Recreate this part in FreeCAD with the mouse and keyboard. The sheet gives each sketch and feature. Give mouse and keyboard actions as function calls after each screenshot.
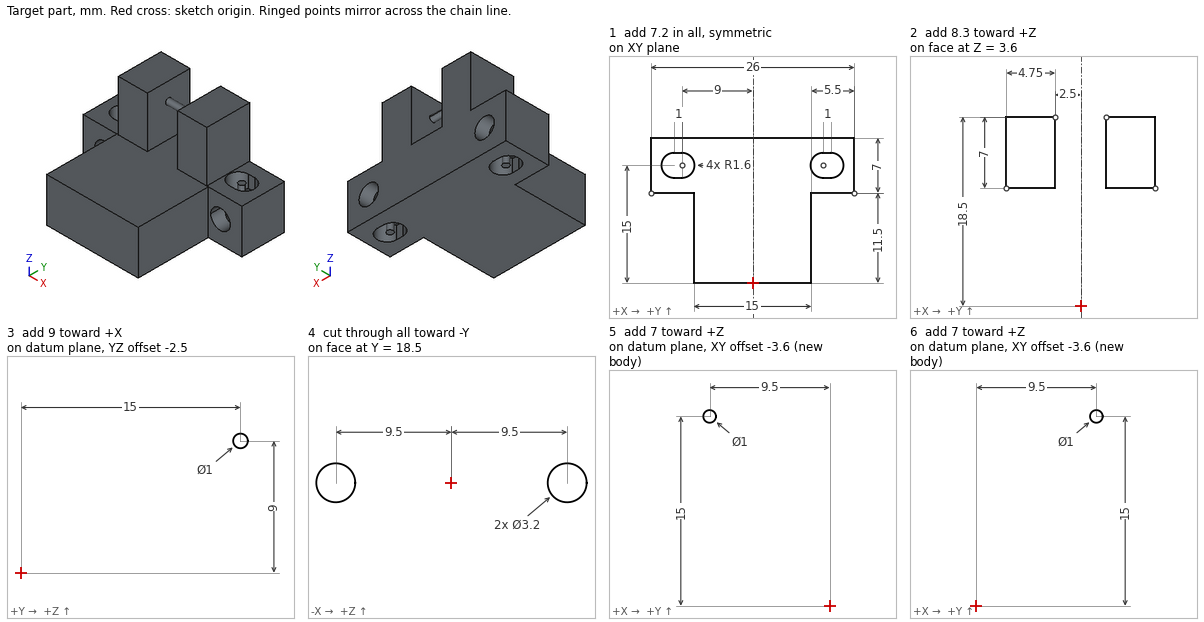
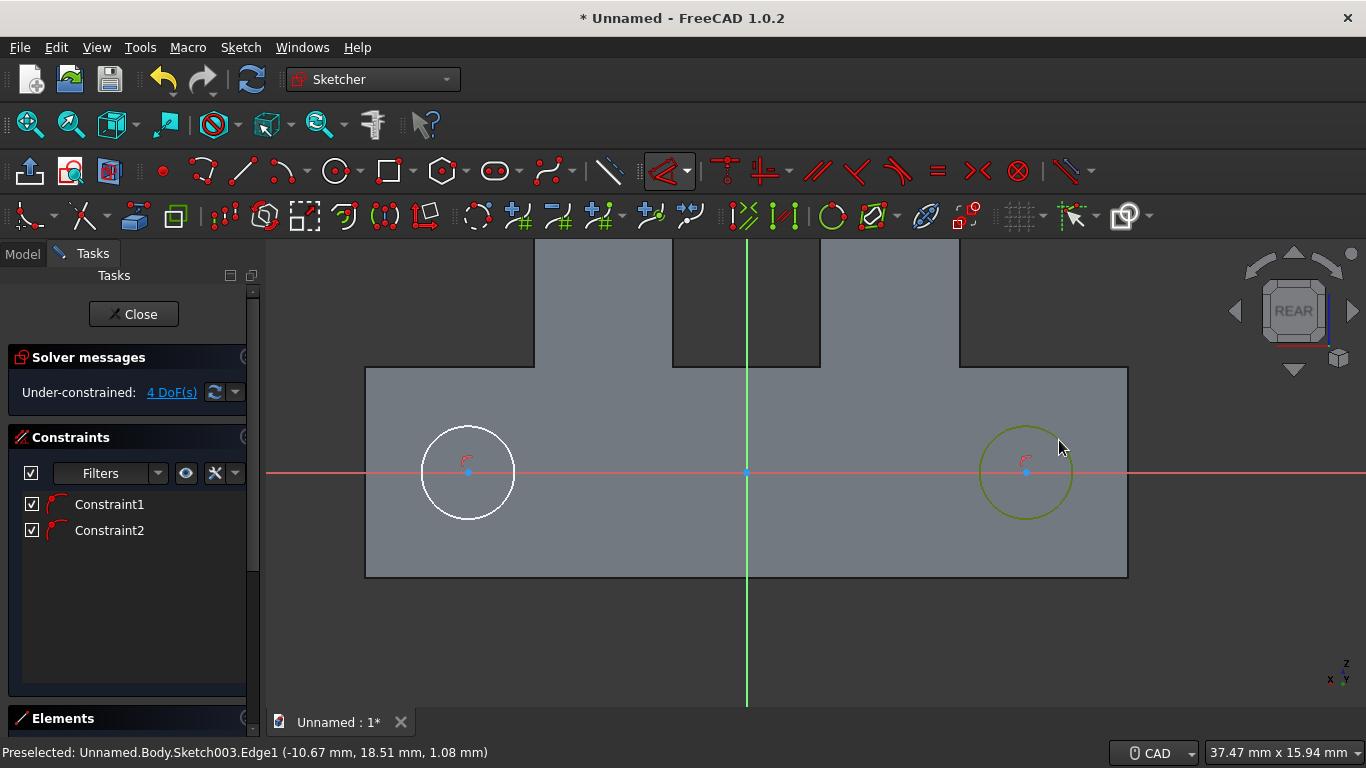
click(501, 440)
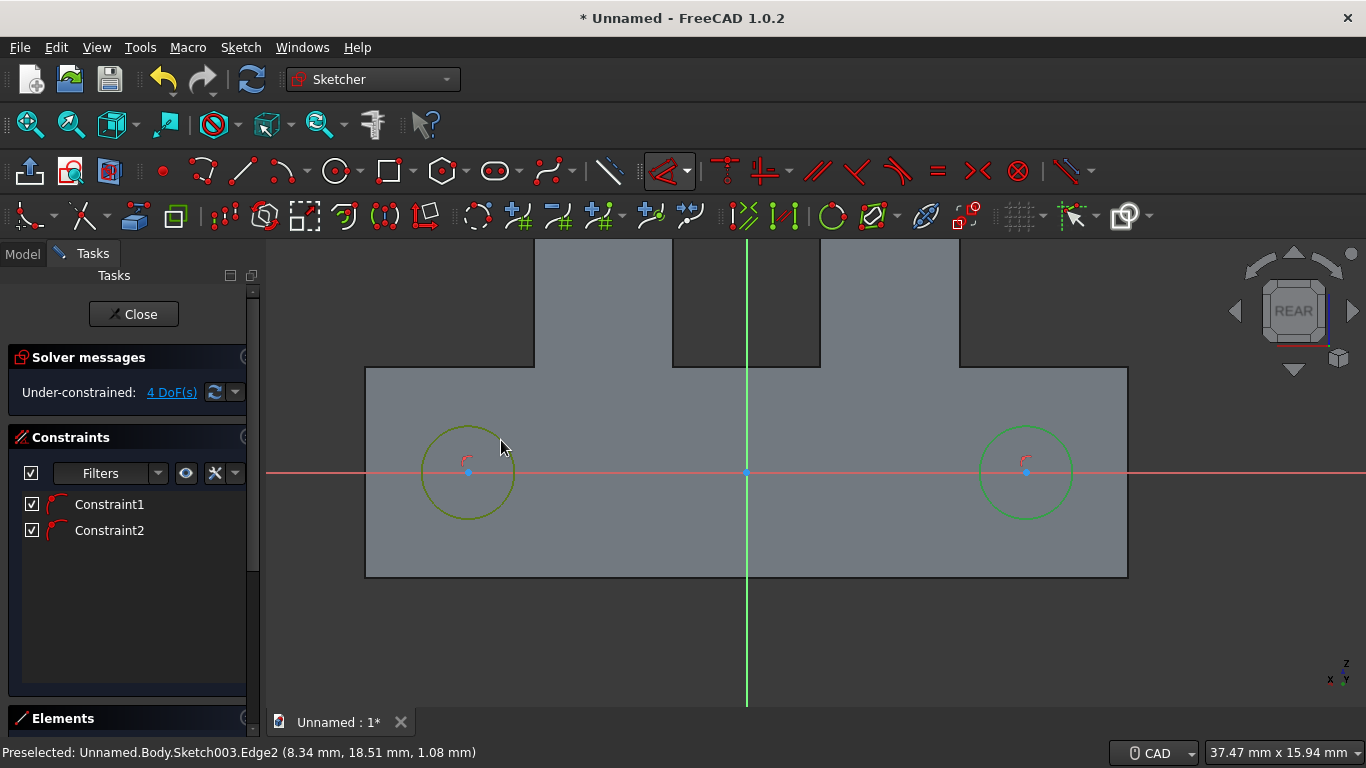
key(e)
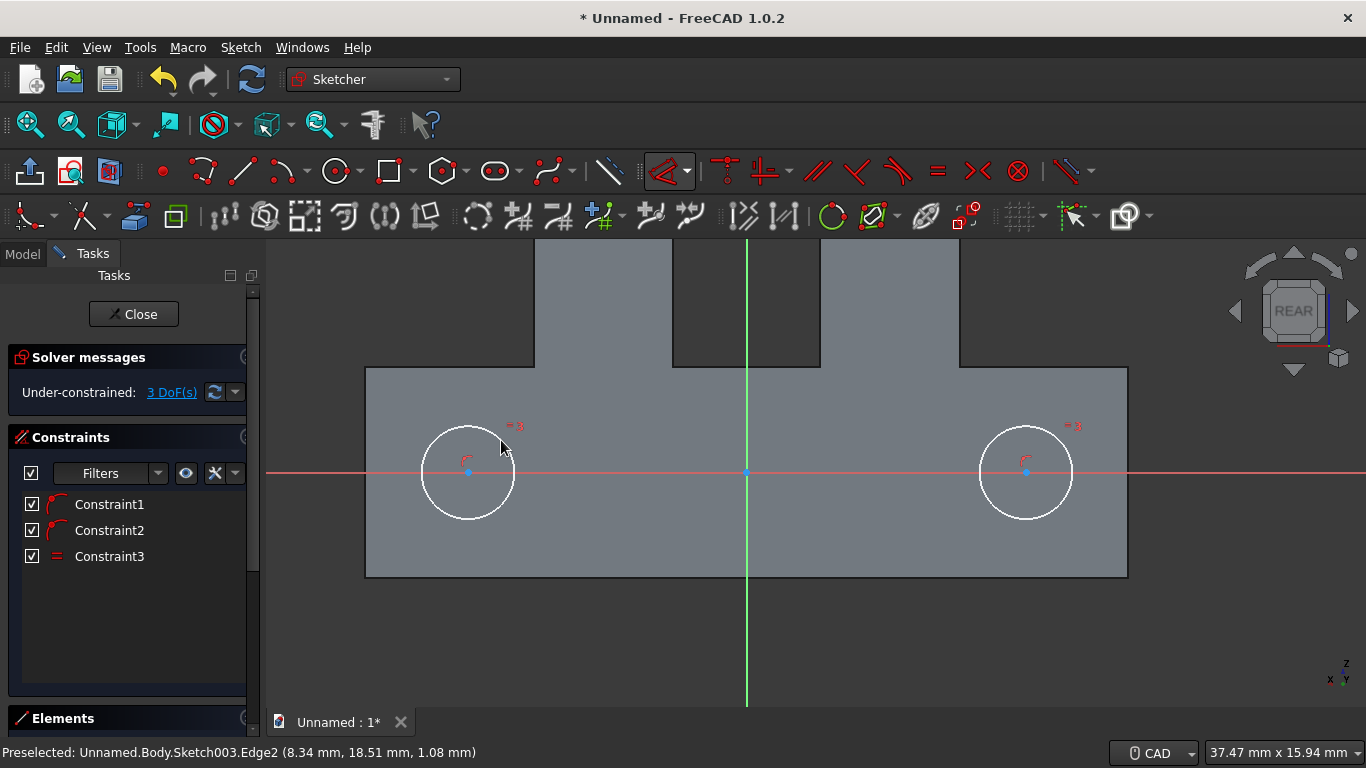
click(1059, 440)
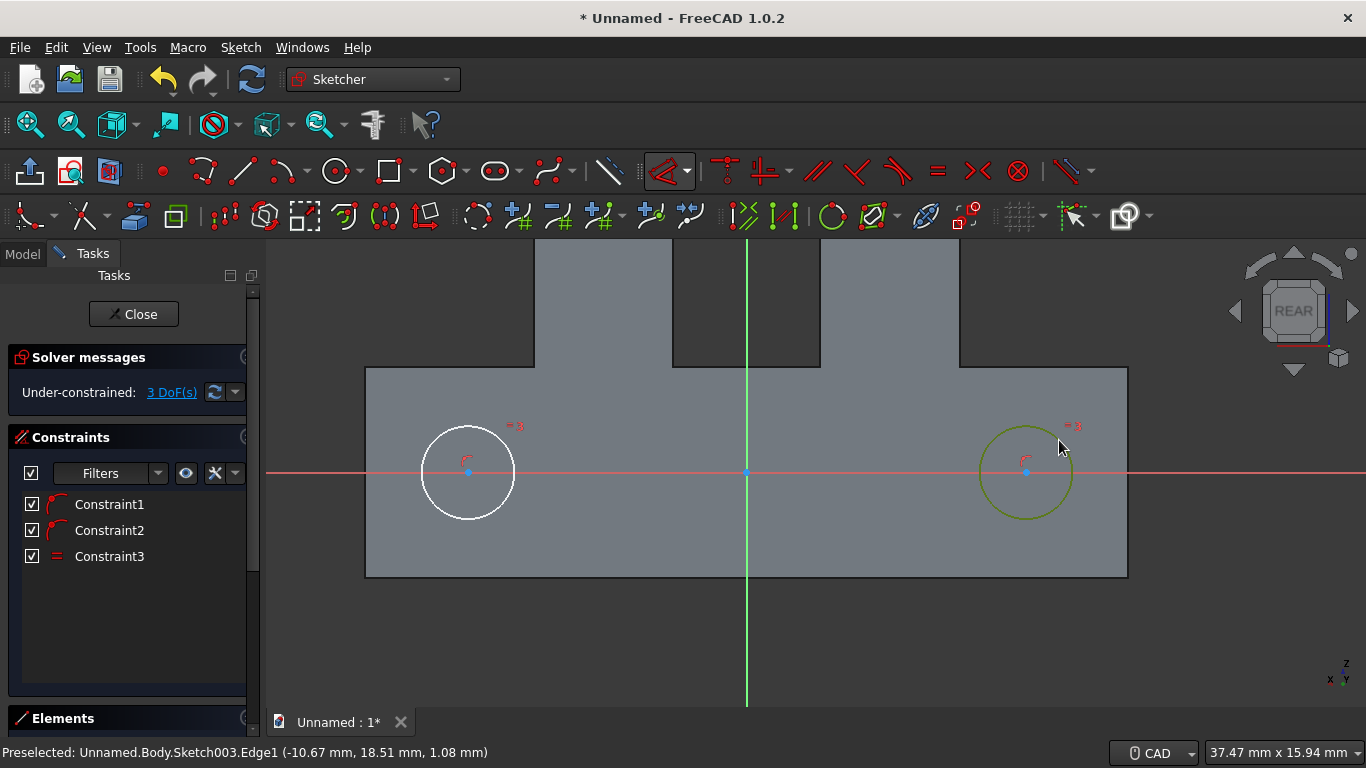
key(k)
key(o)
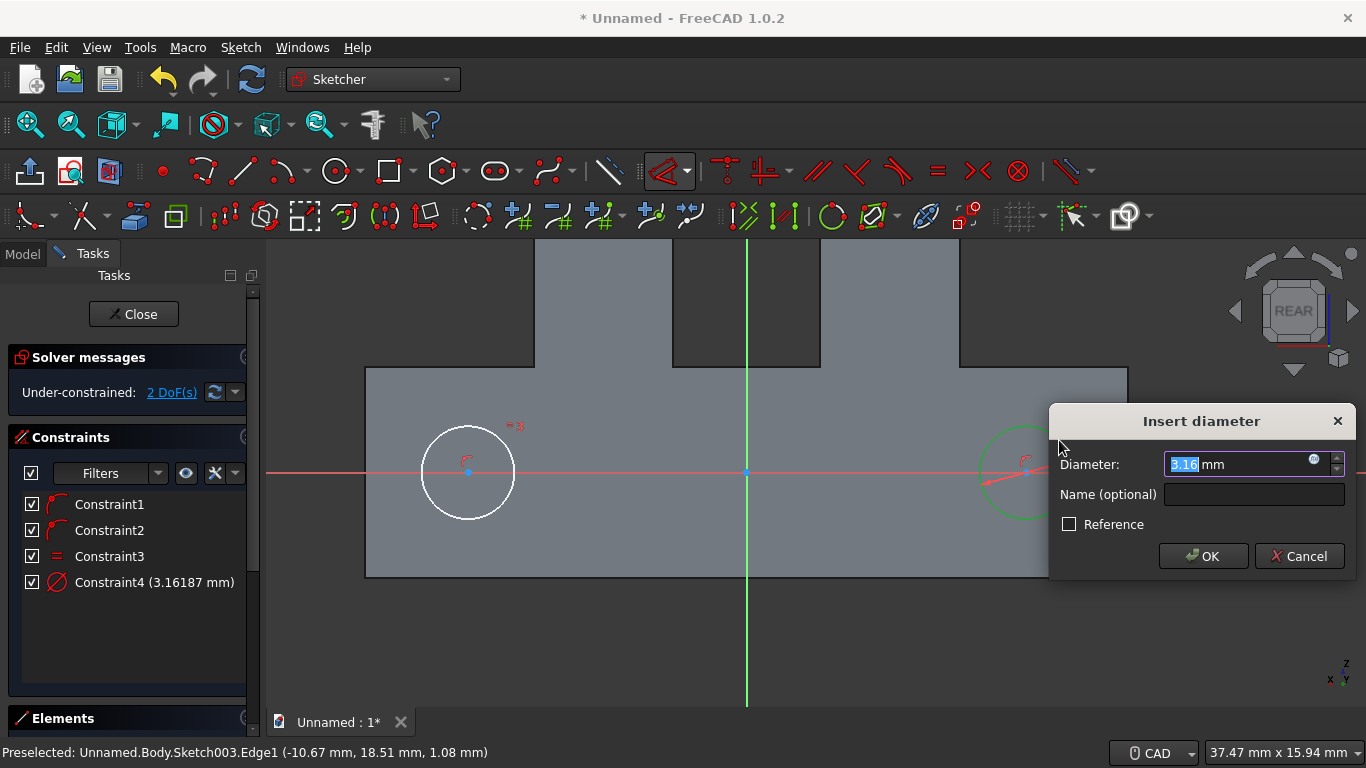
text(3.2)
key(Return)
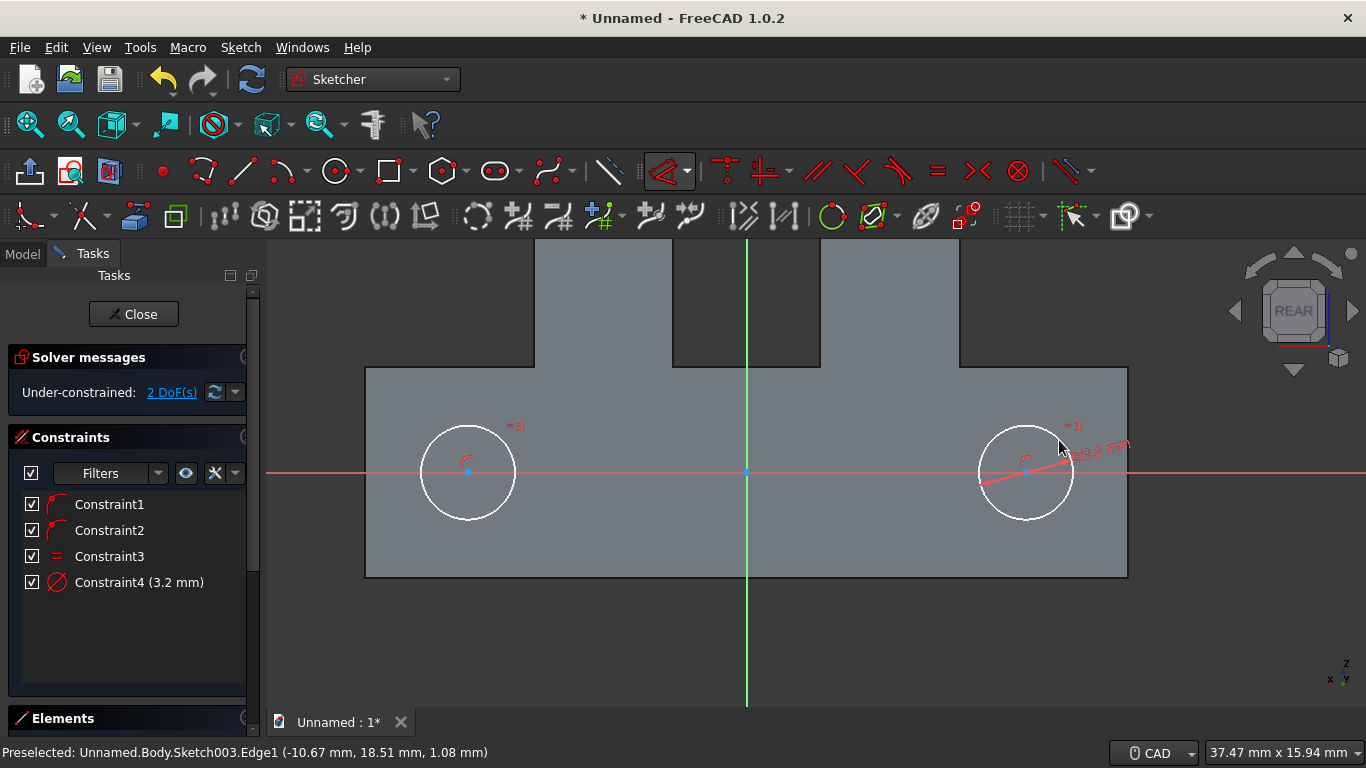
click(1026, 473)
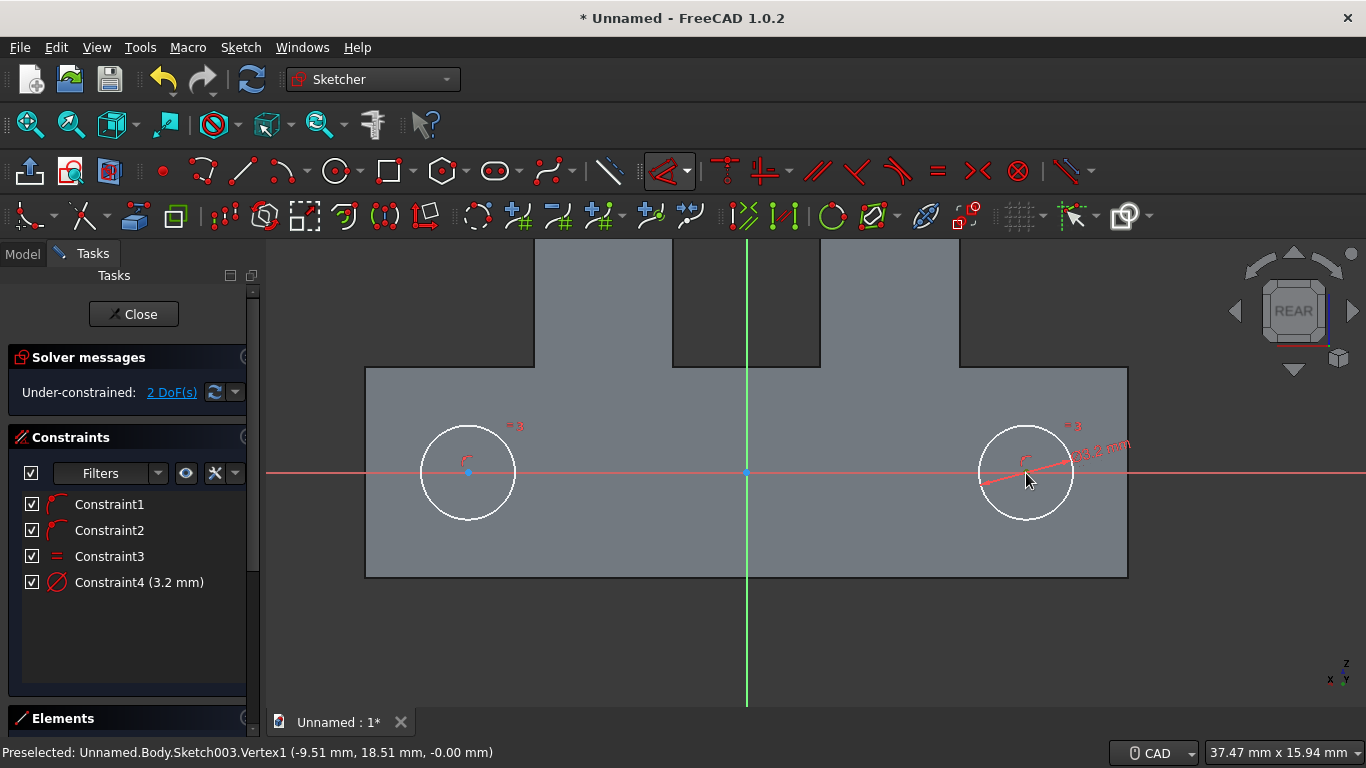
key(l)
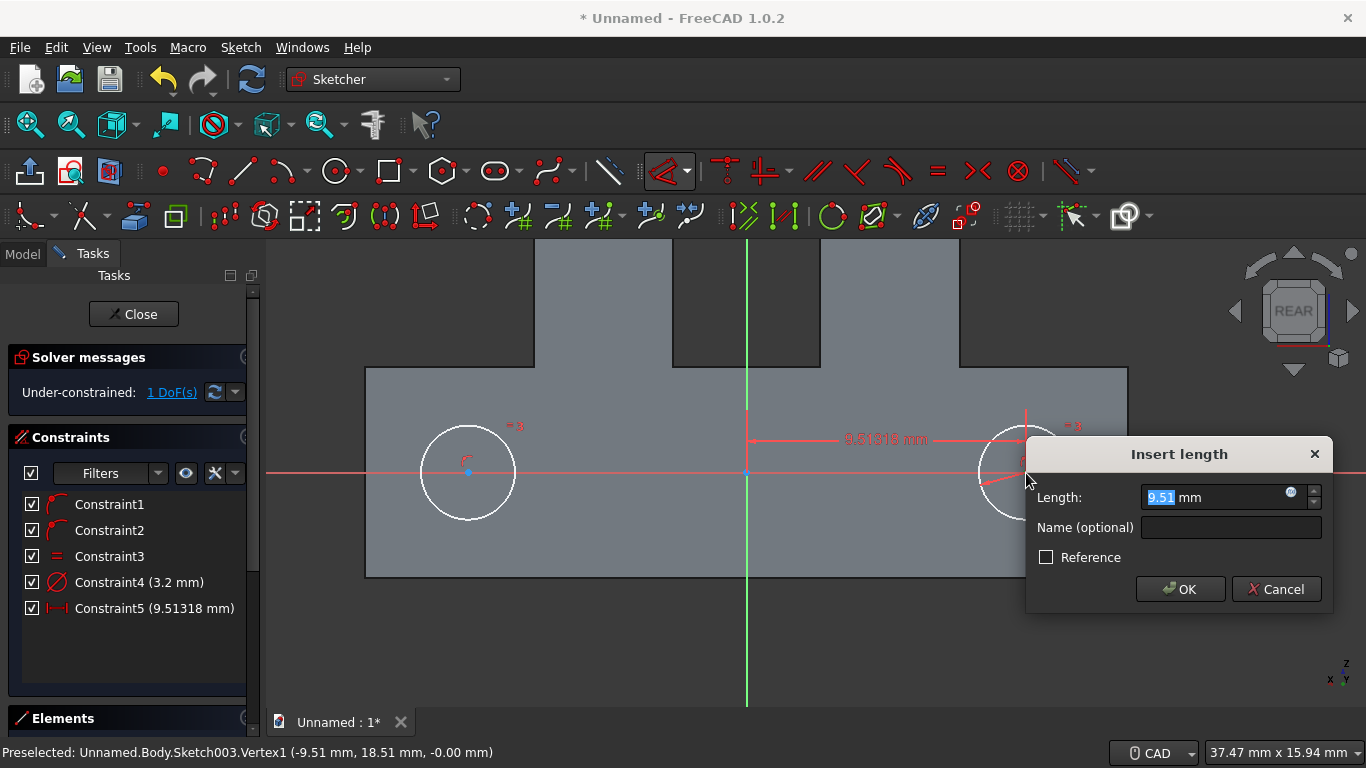
text(9.5)
key(Return)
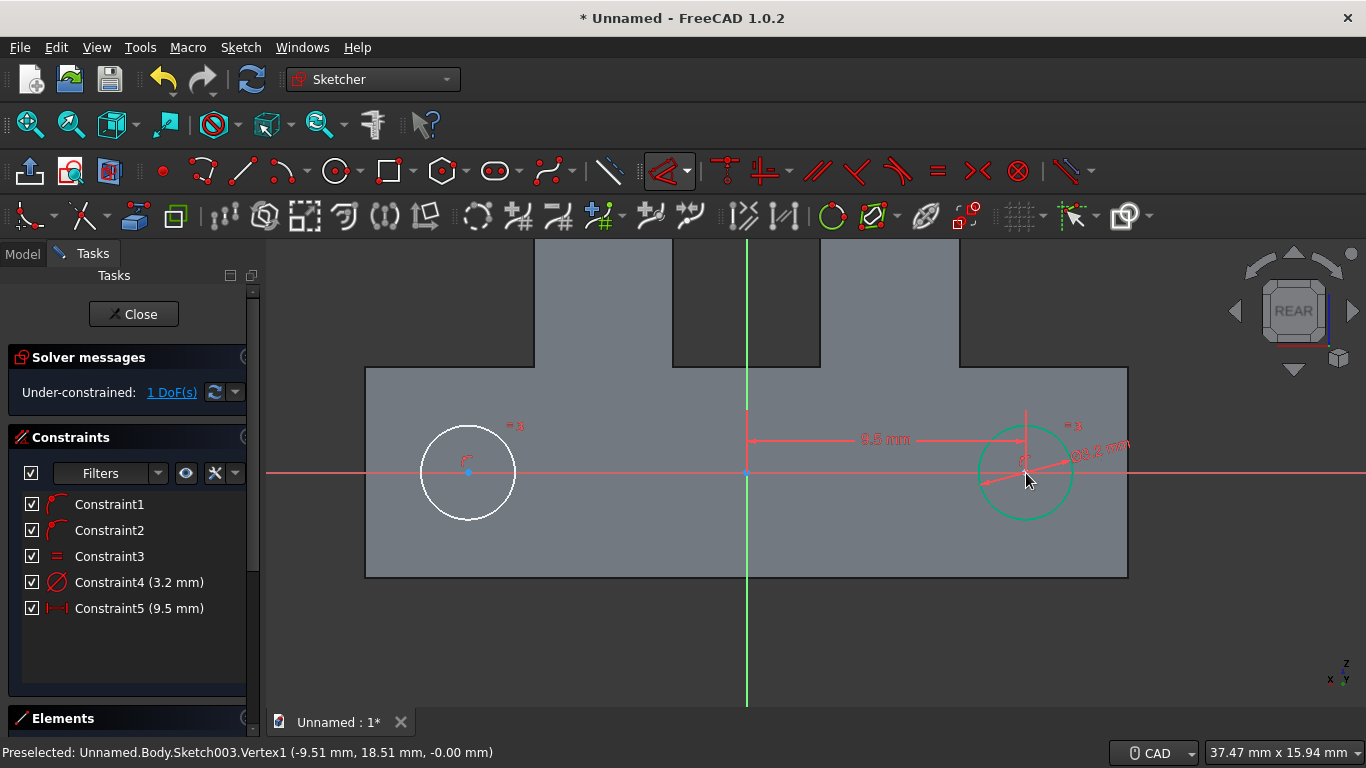
click(468, 473)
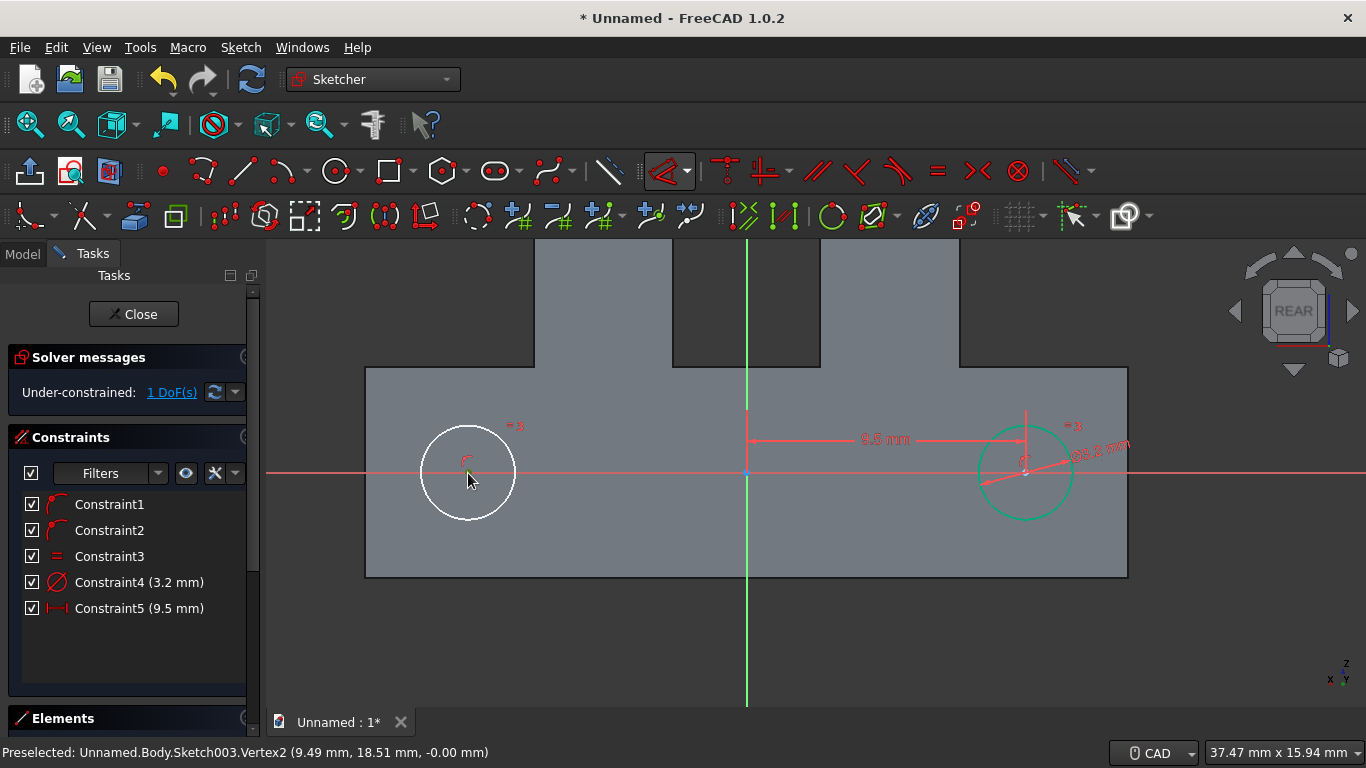
key(l)